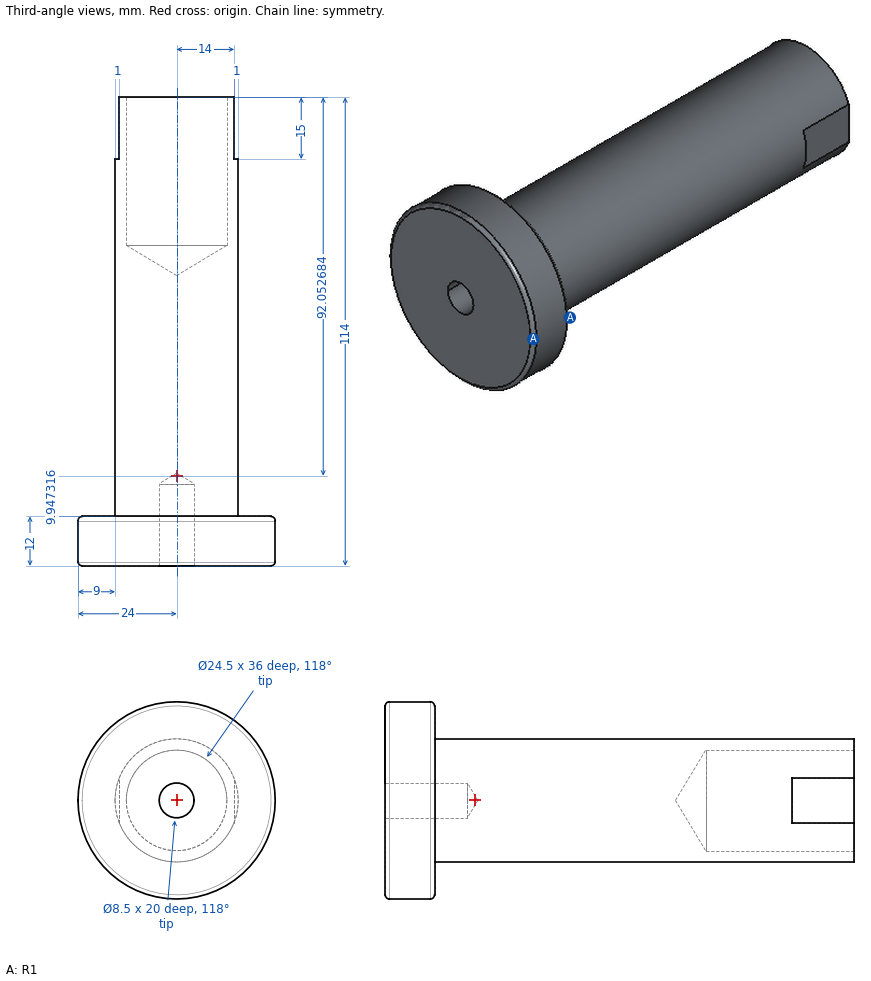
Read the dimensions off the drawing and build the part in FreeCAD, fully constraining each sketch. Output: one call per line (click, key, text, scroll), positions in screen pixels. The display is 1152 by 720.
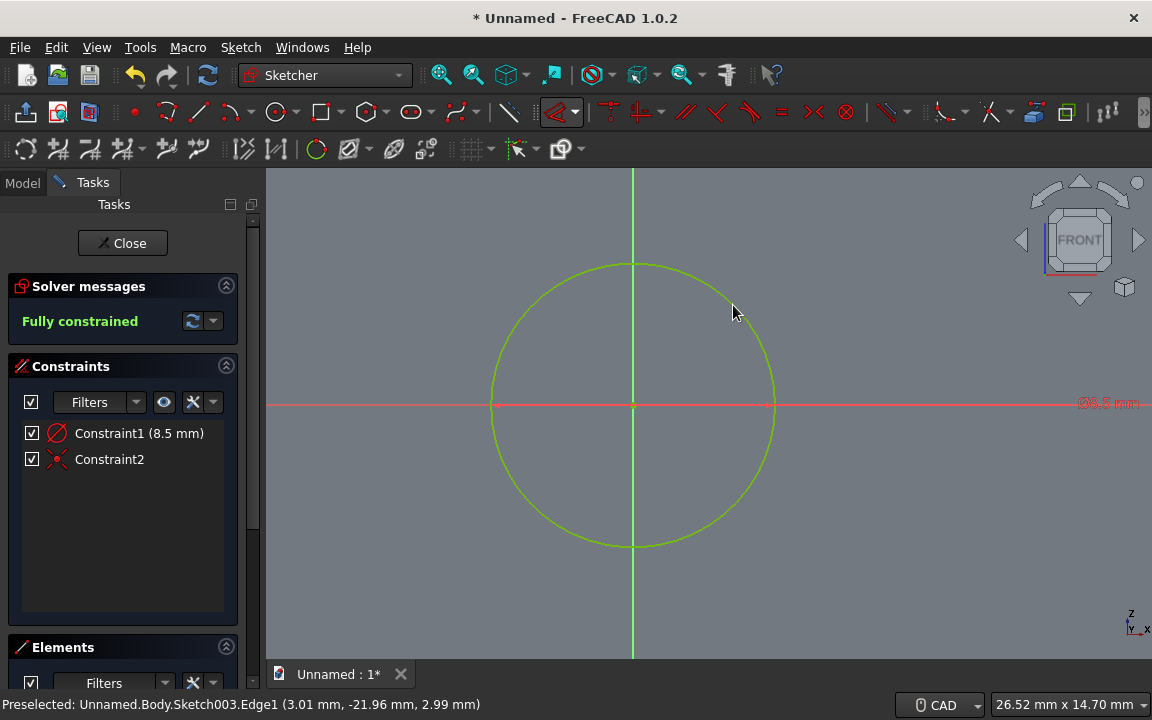
click(123, 243)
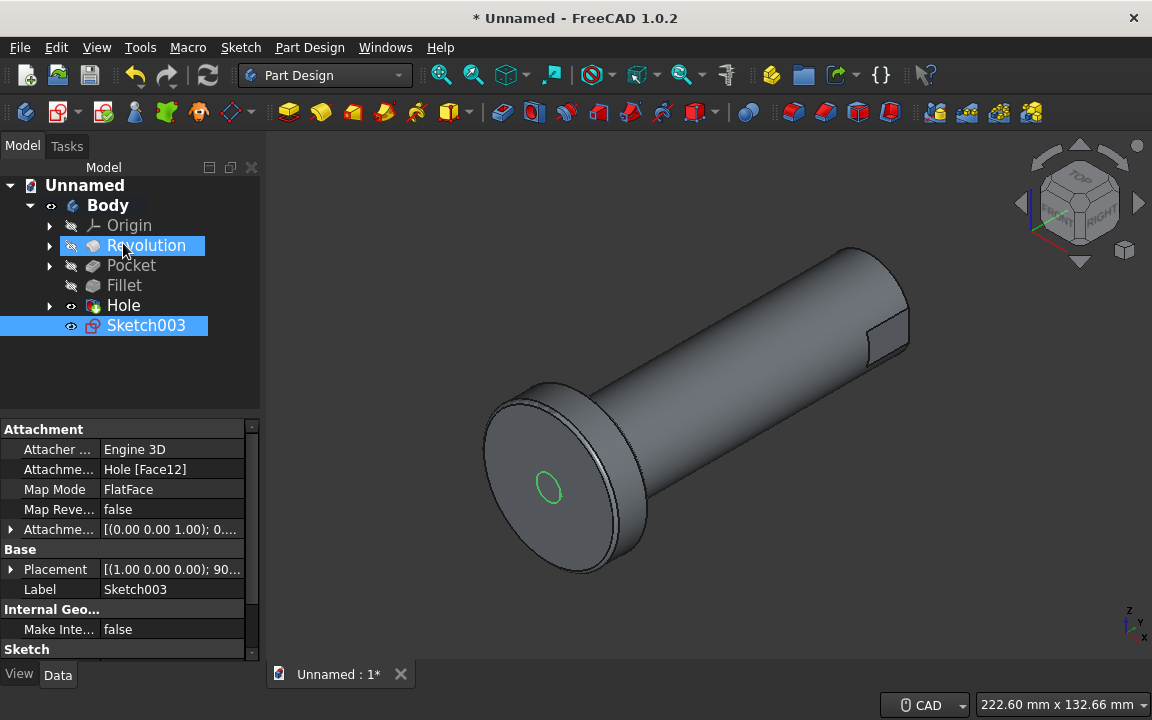
click(536, 112)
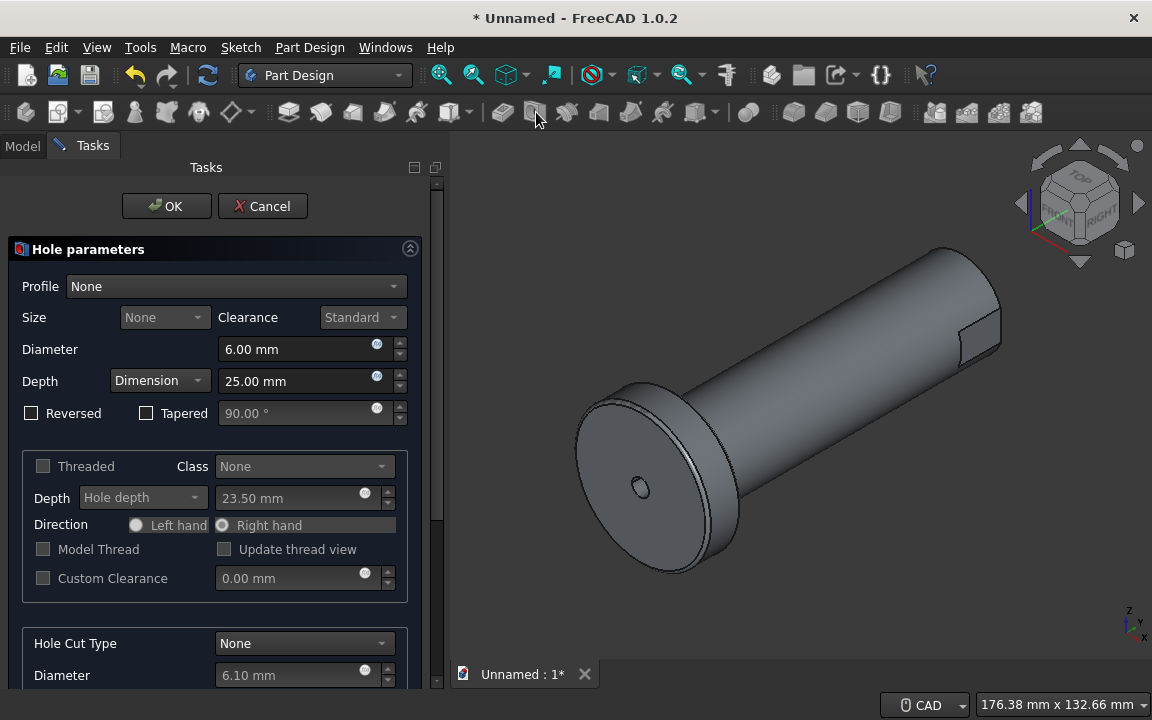
triple_click(305, 349)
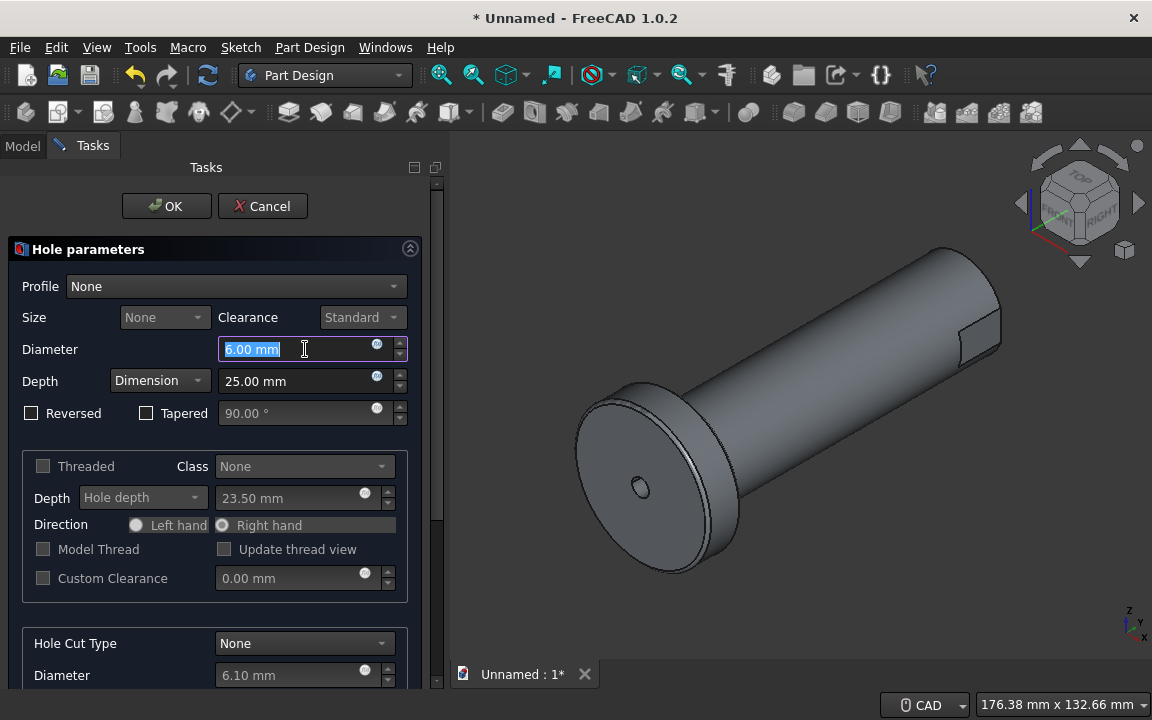
text(8.5)
key(Tab)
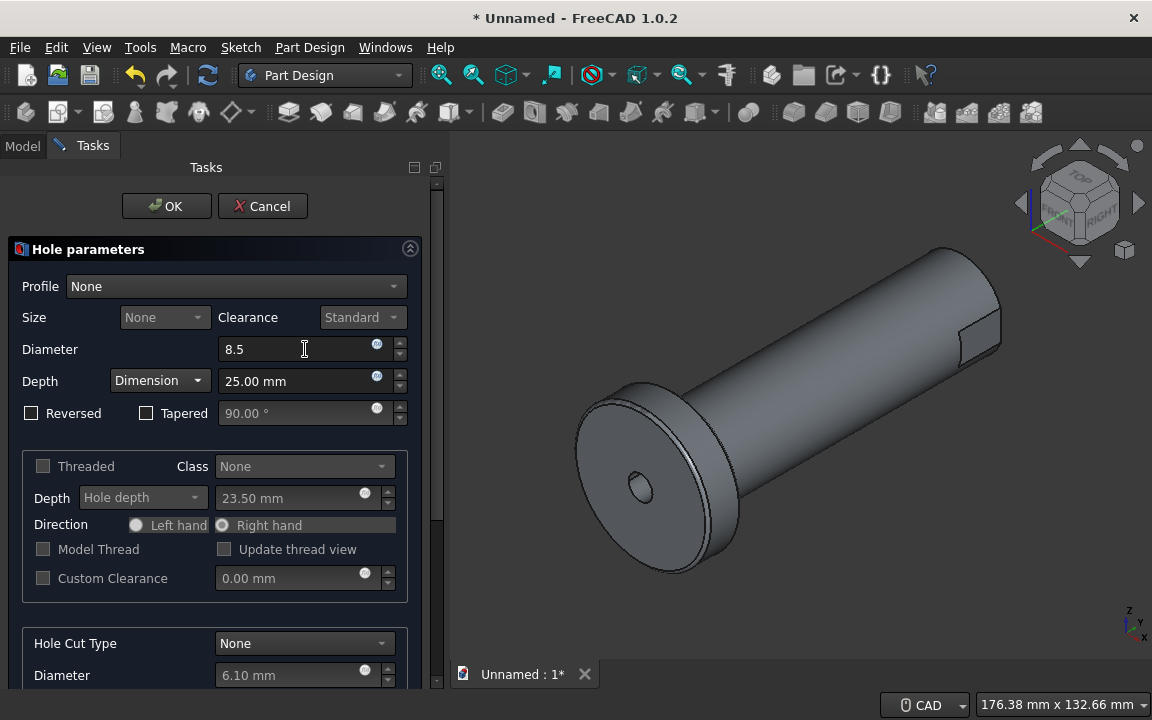
triple_click(305, 381)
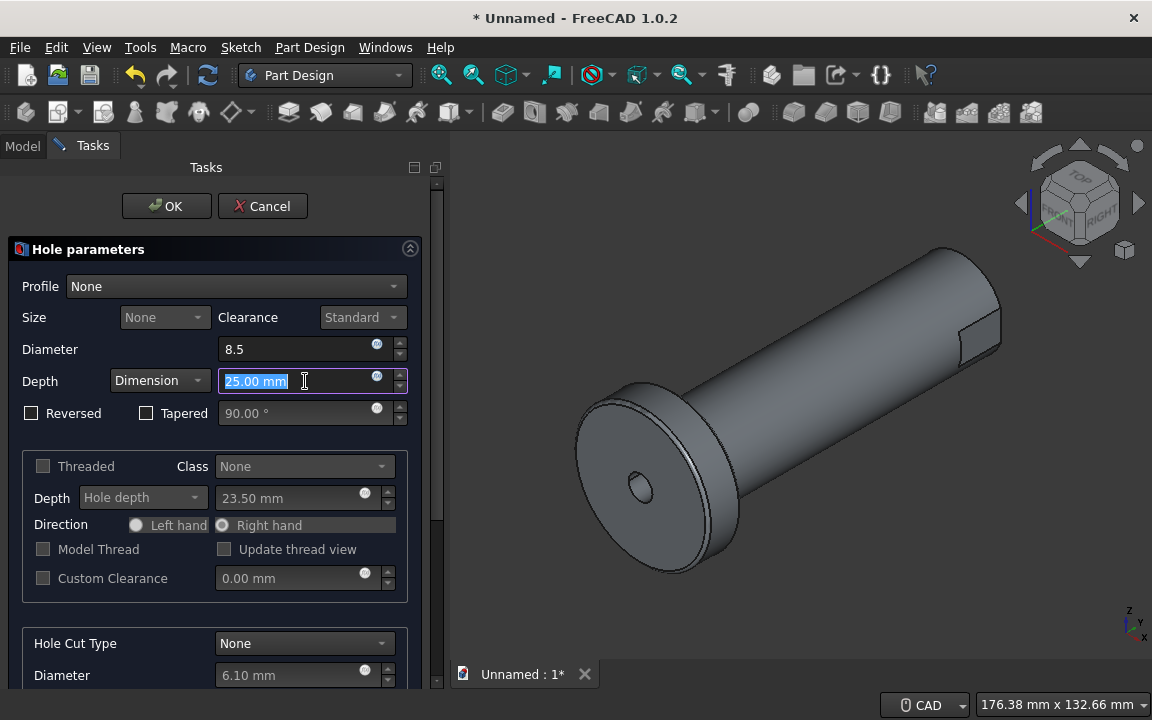
text(20)
key(Tab)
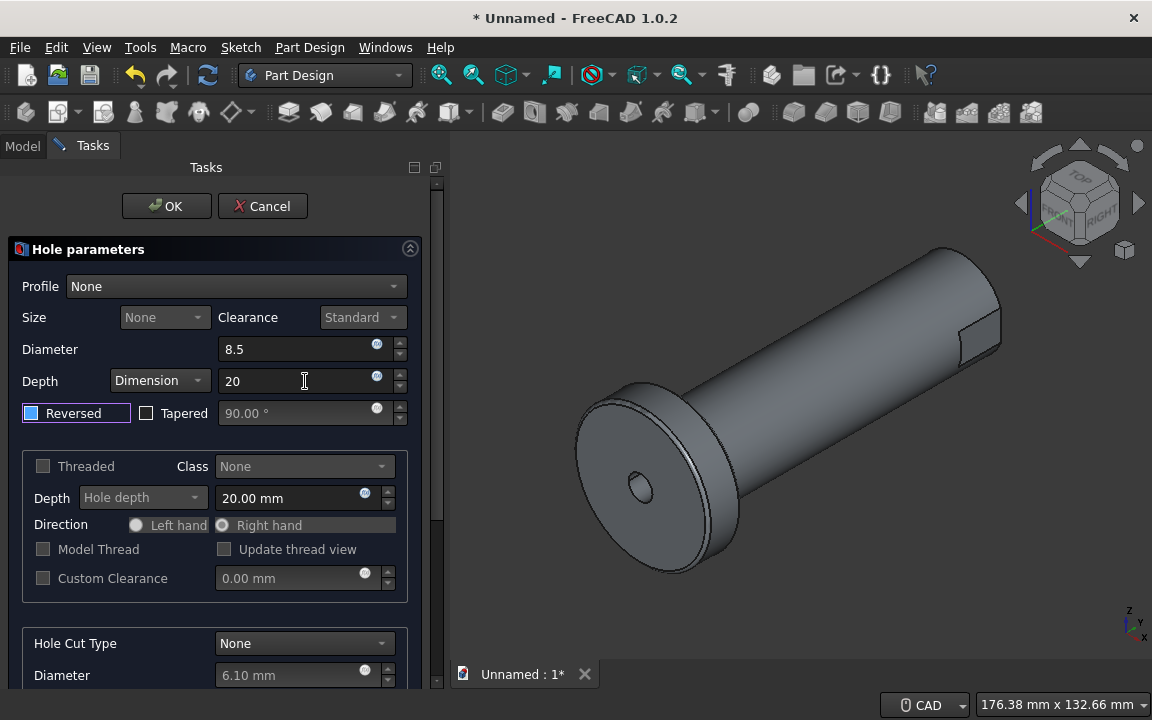
click(167, 206)